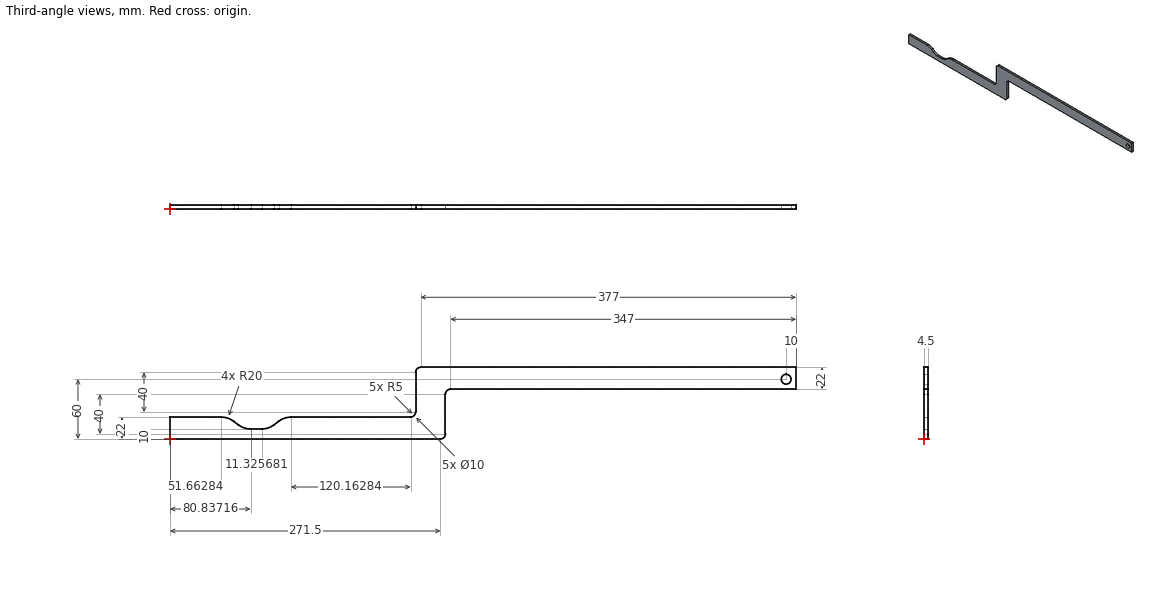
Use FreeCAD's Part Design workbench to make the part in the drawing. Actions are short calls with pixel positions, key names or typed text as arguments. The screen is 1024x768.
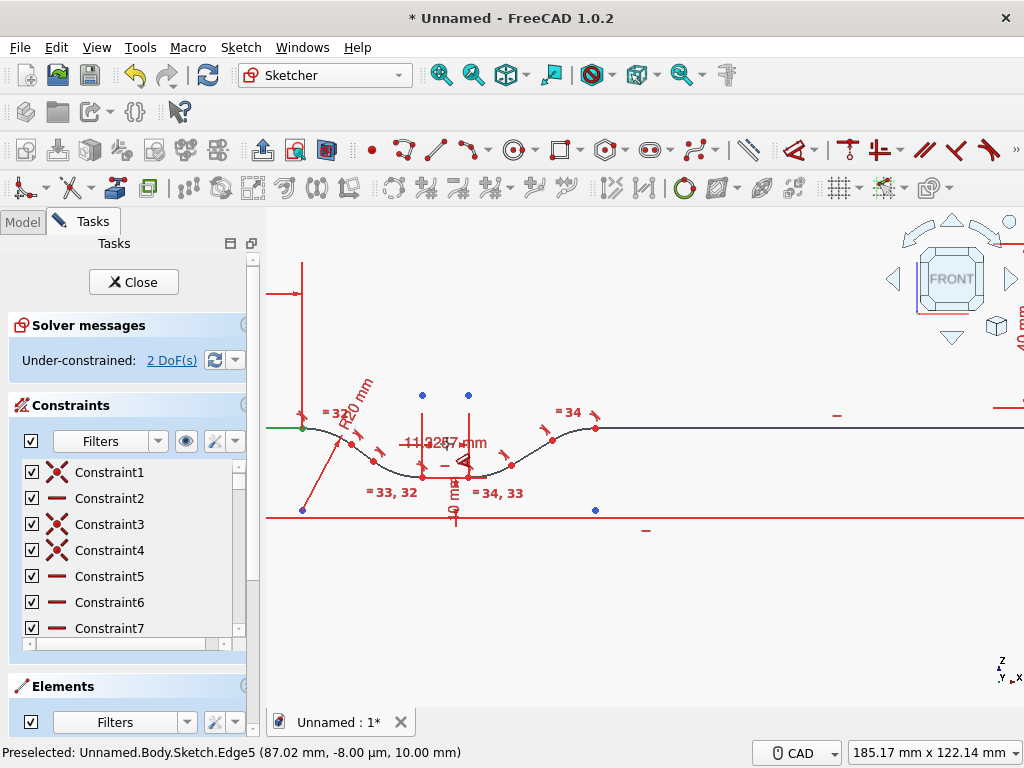
scroll(418, 474, down, 9)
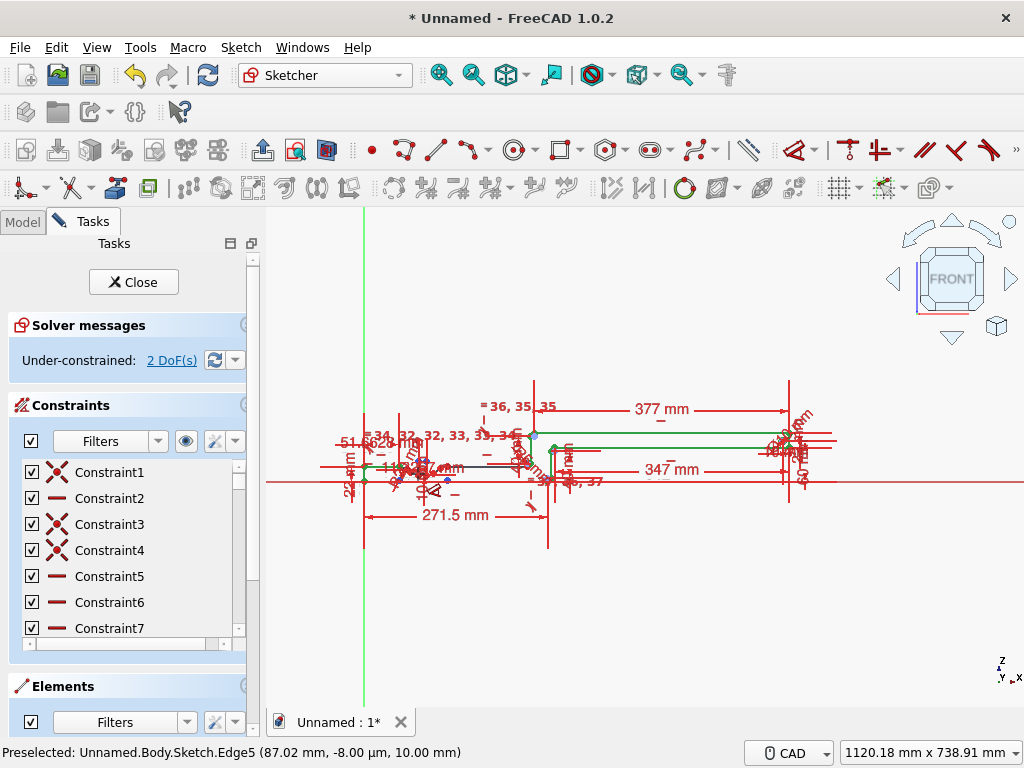
click(471, 467)
click(487, 409)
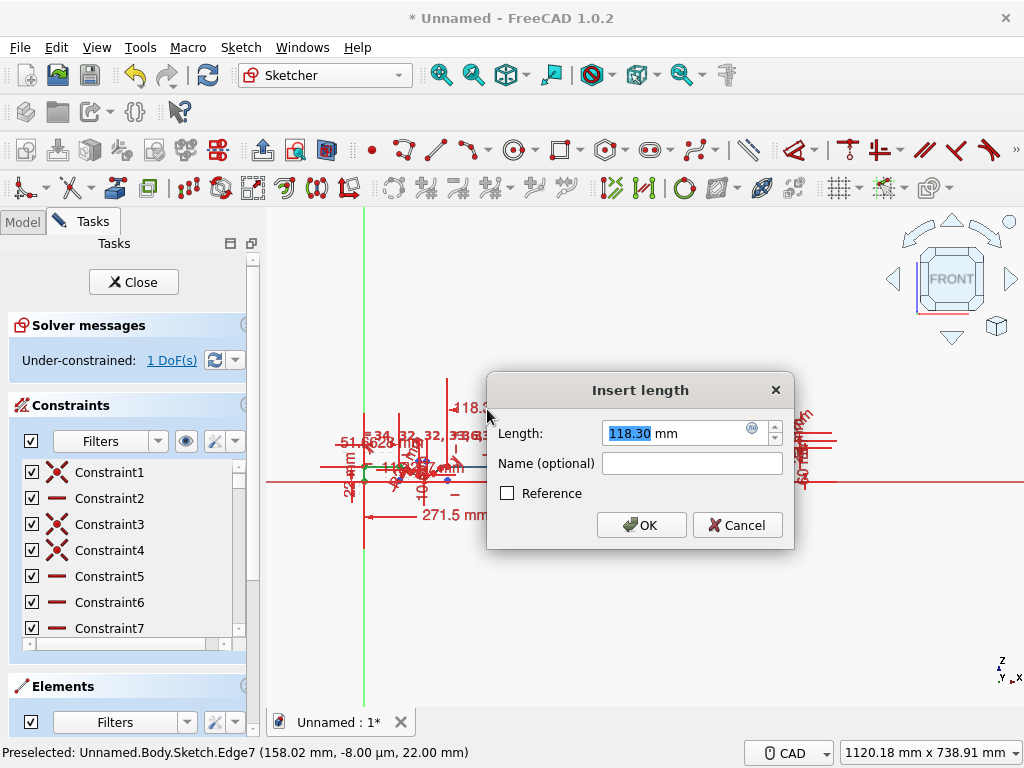
text(120.16284)
key(Return)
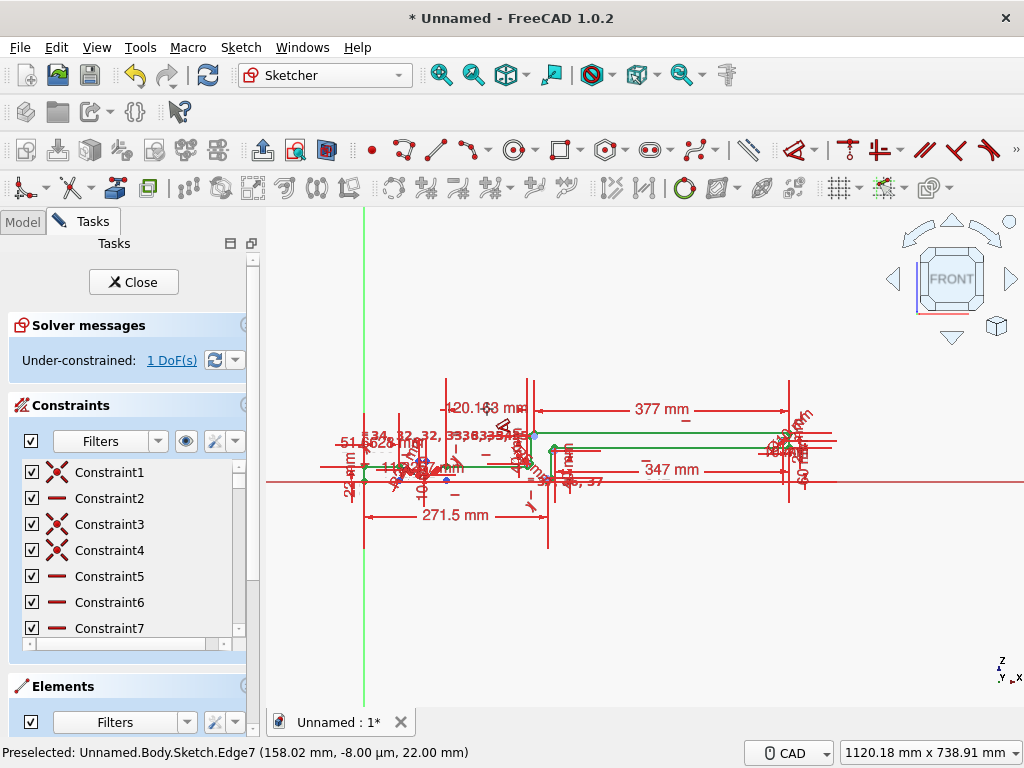
scroll(419, 475, up, 3)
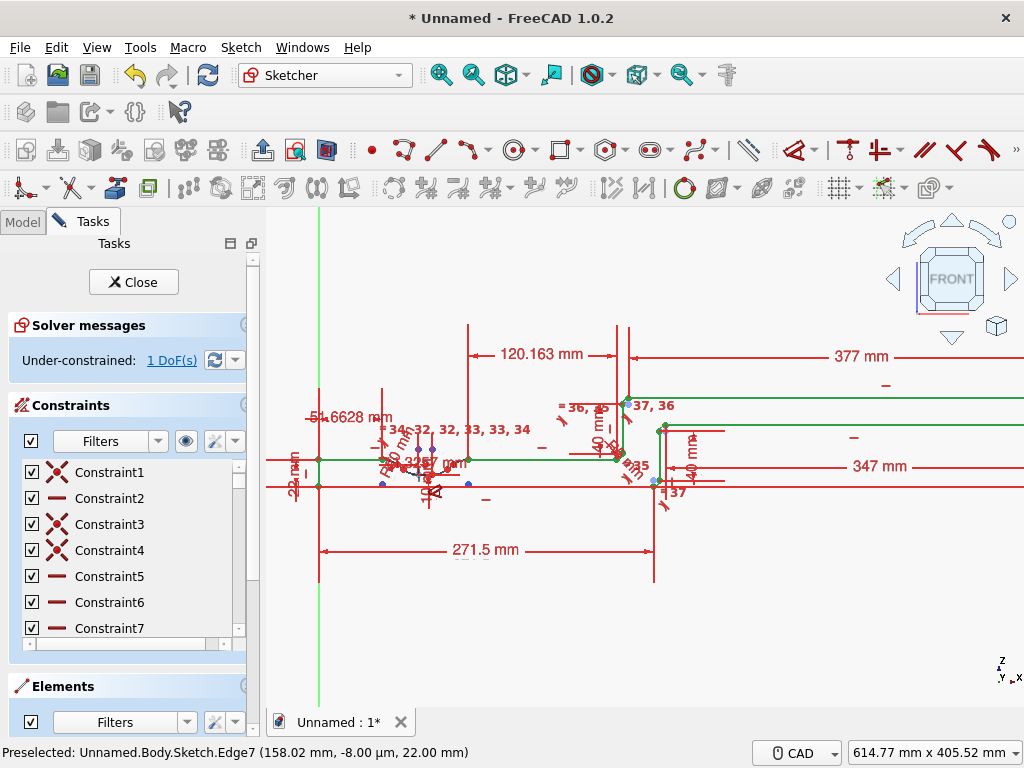
click(418, 475)
click(369, 521)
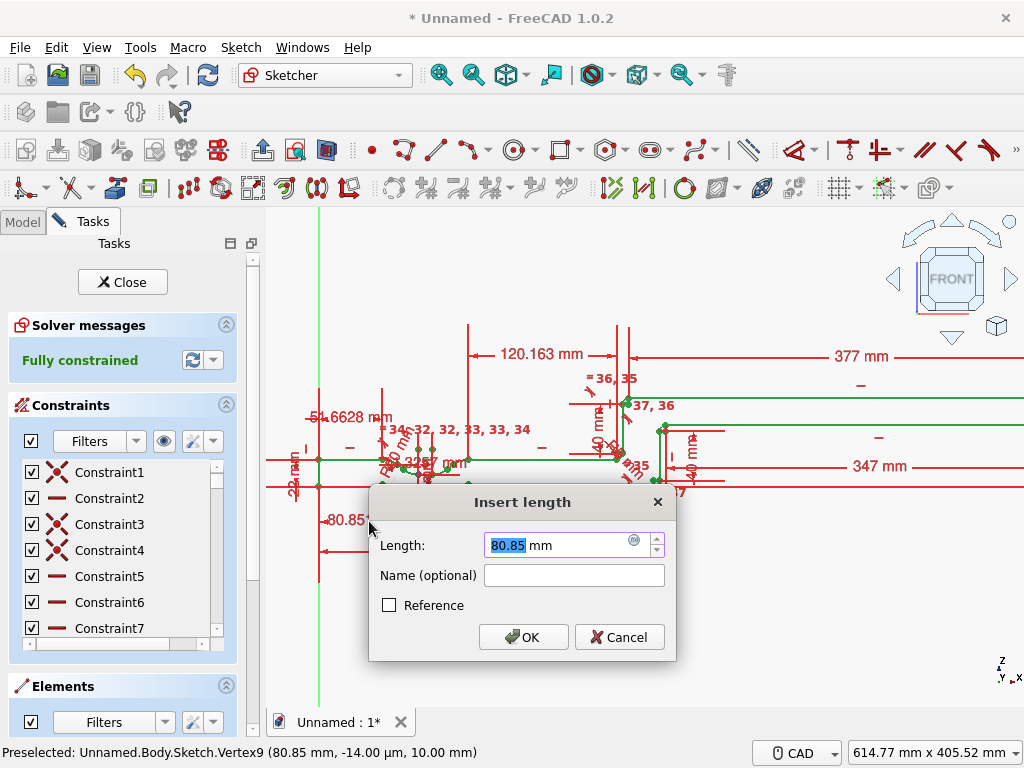
text(80.83716)
key(Return)
key(Escape)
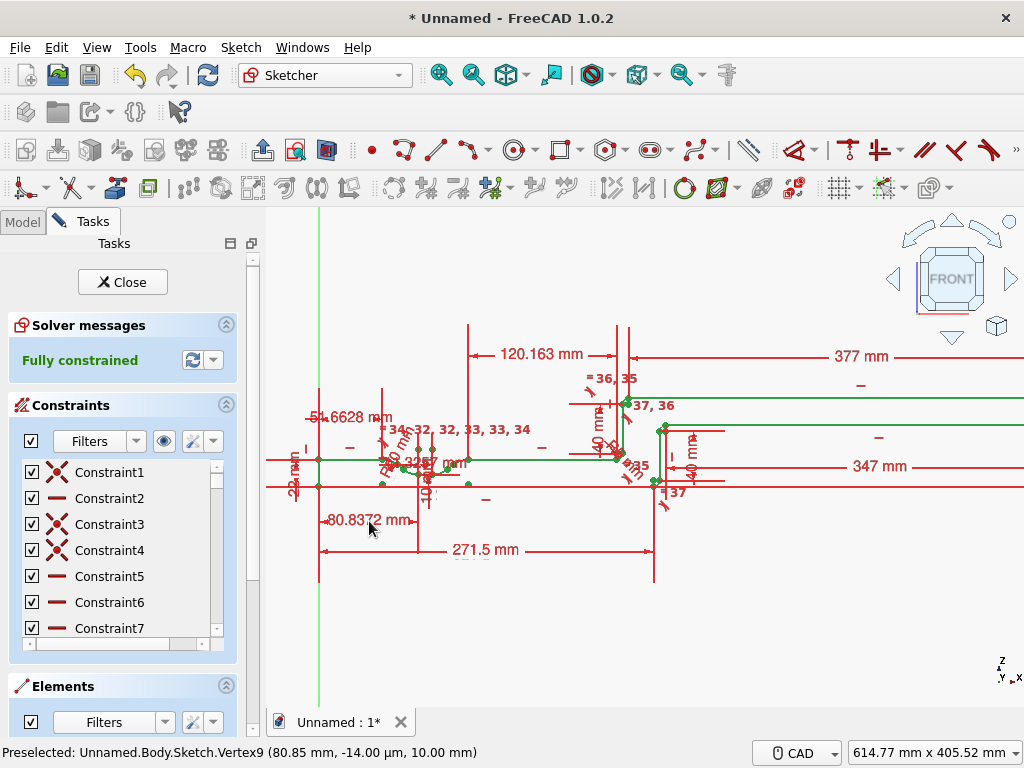
click(123, 282)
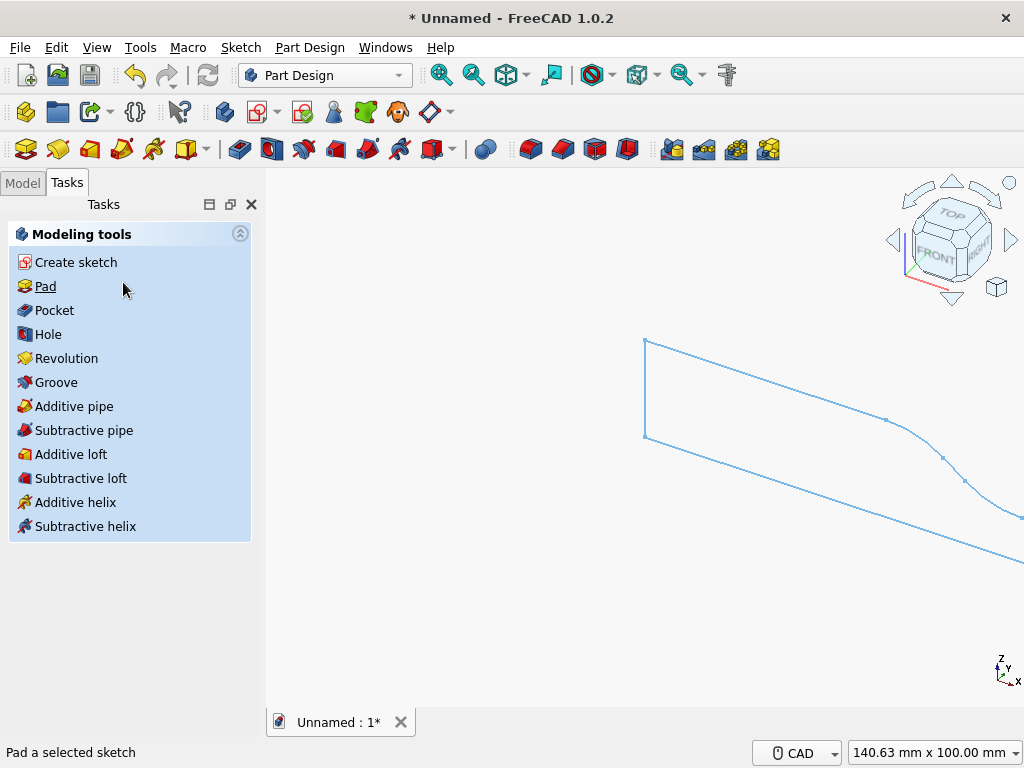
click(26, 150)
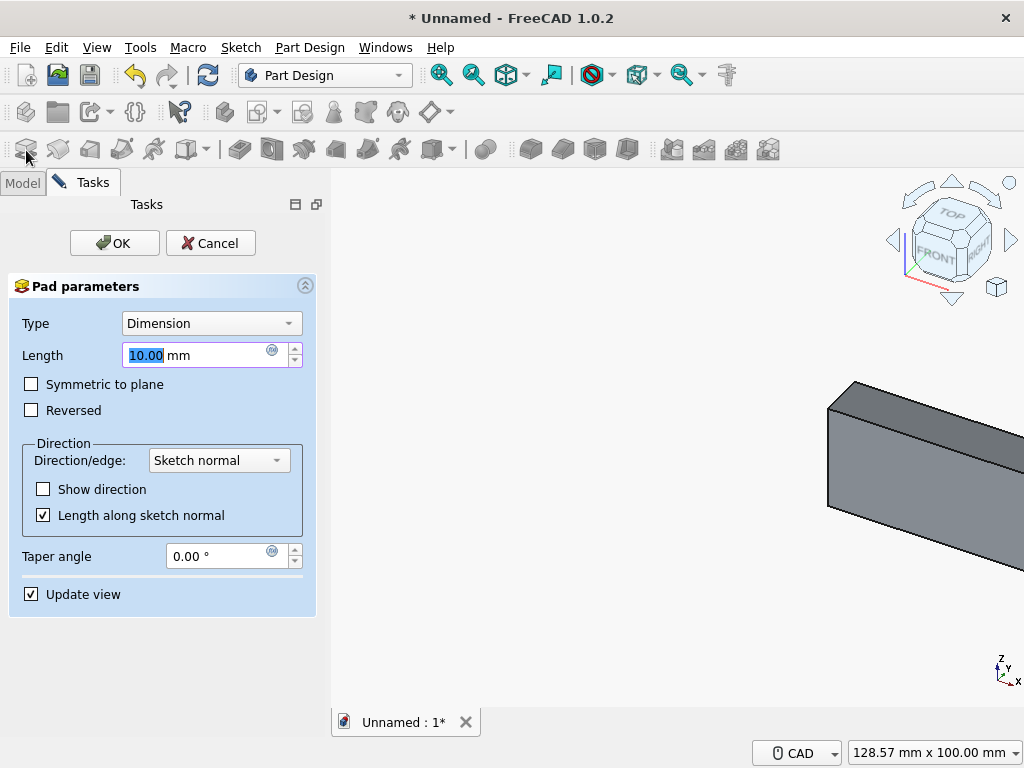
text(4.5)
key(Tab)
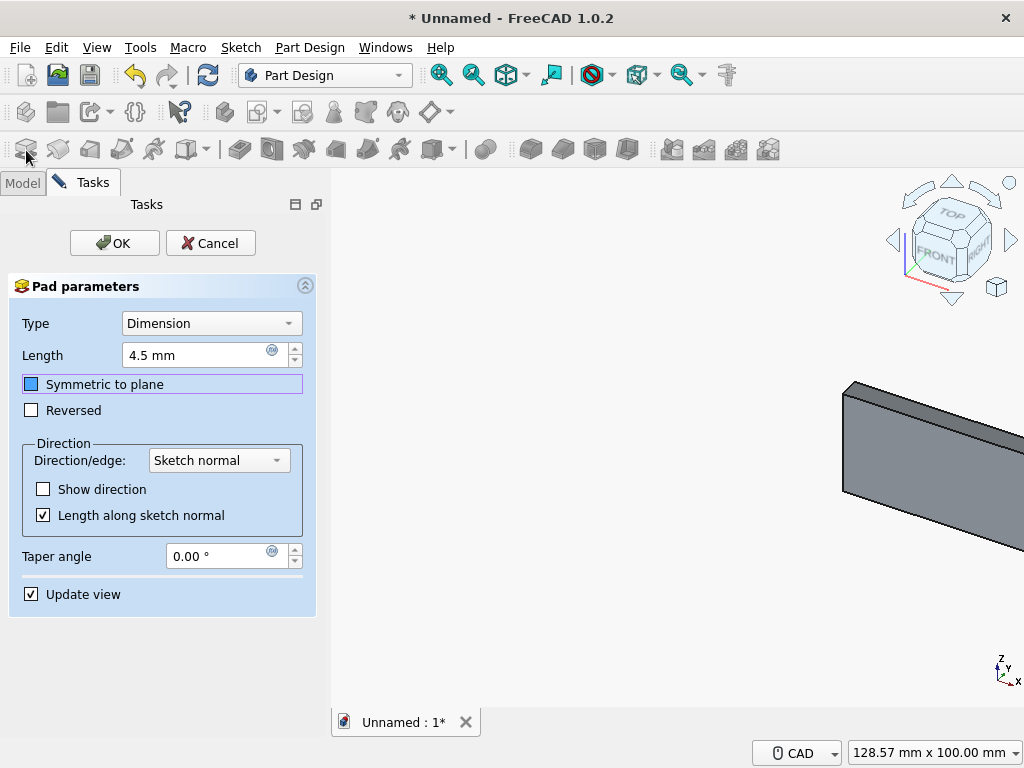
click(30, 410)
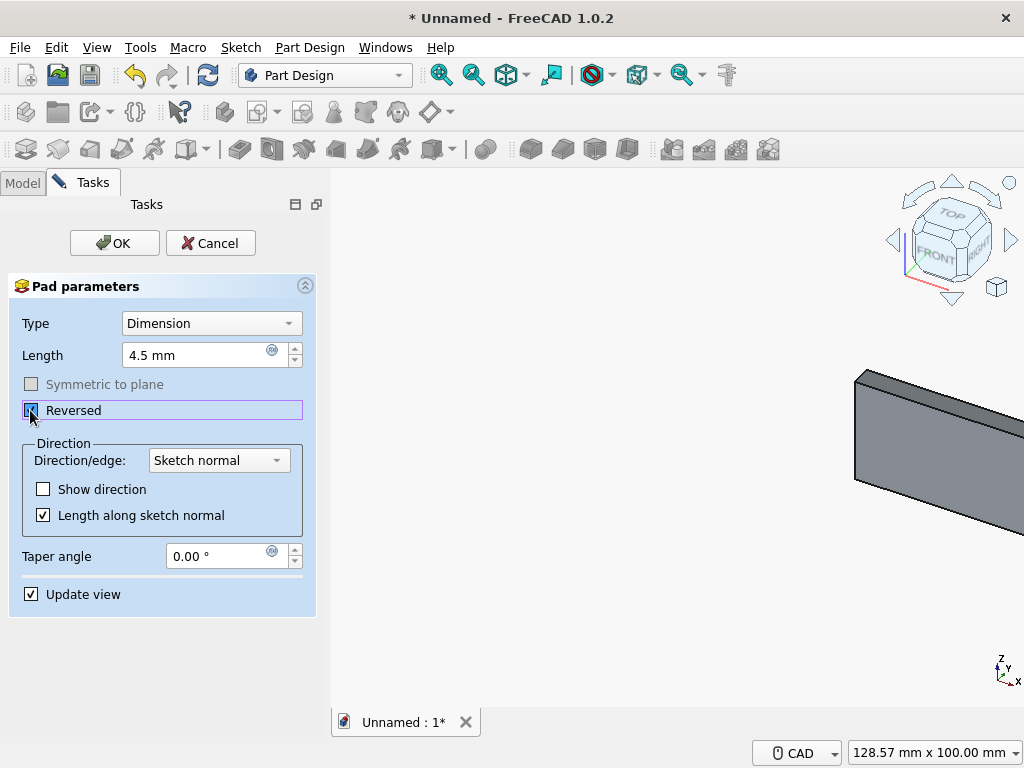
click(115, 243)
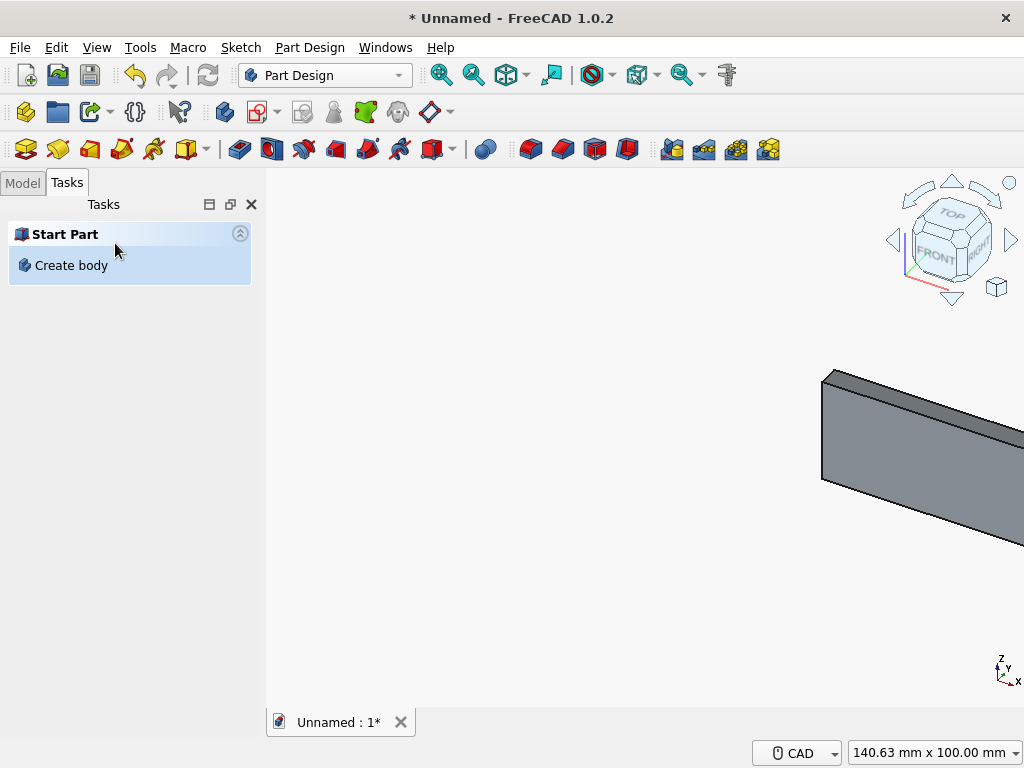
key(0)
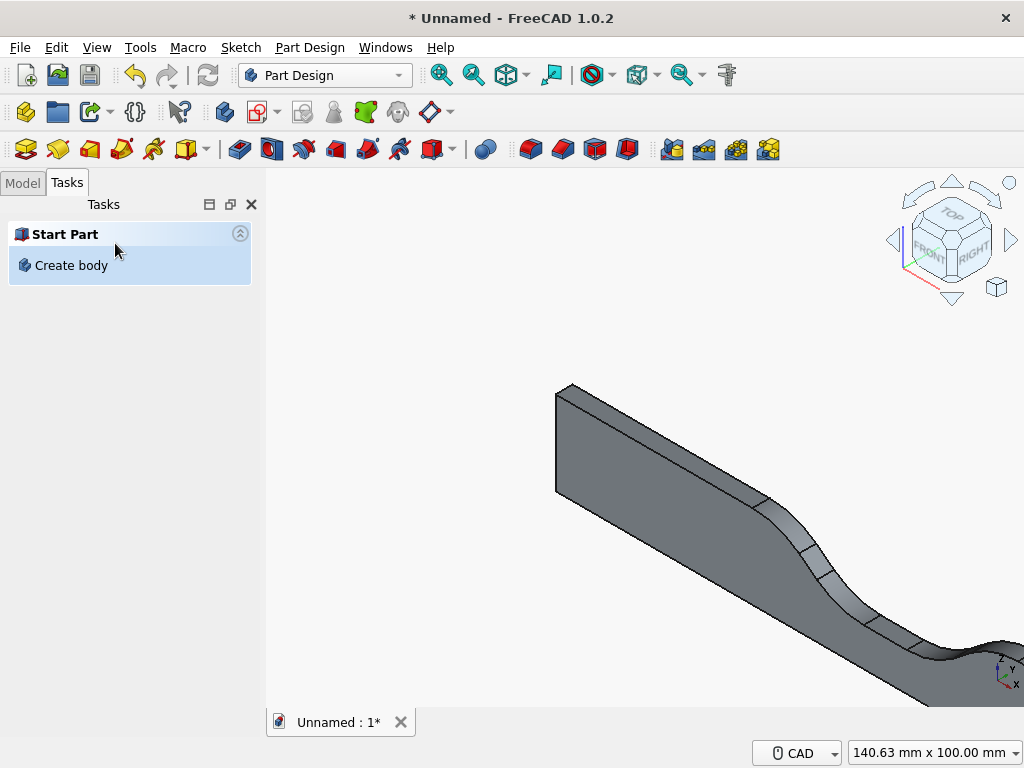
key(v)
key(f)